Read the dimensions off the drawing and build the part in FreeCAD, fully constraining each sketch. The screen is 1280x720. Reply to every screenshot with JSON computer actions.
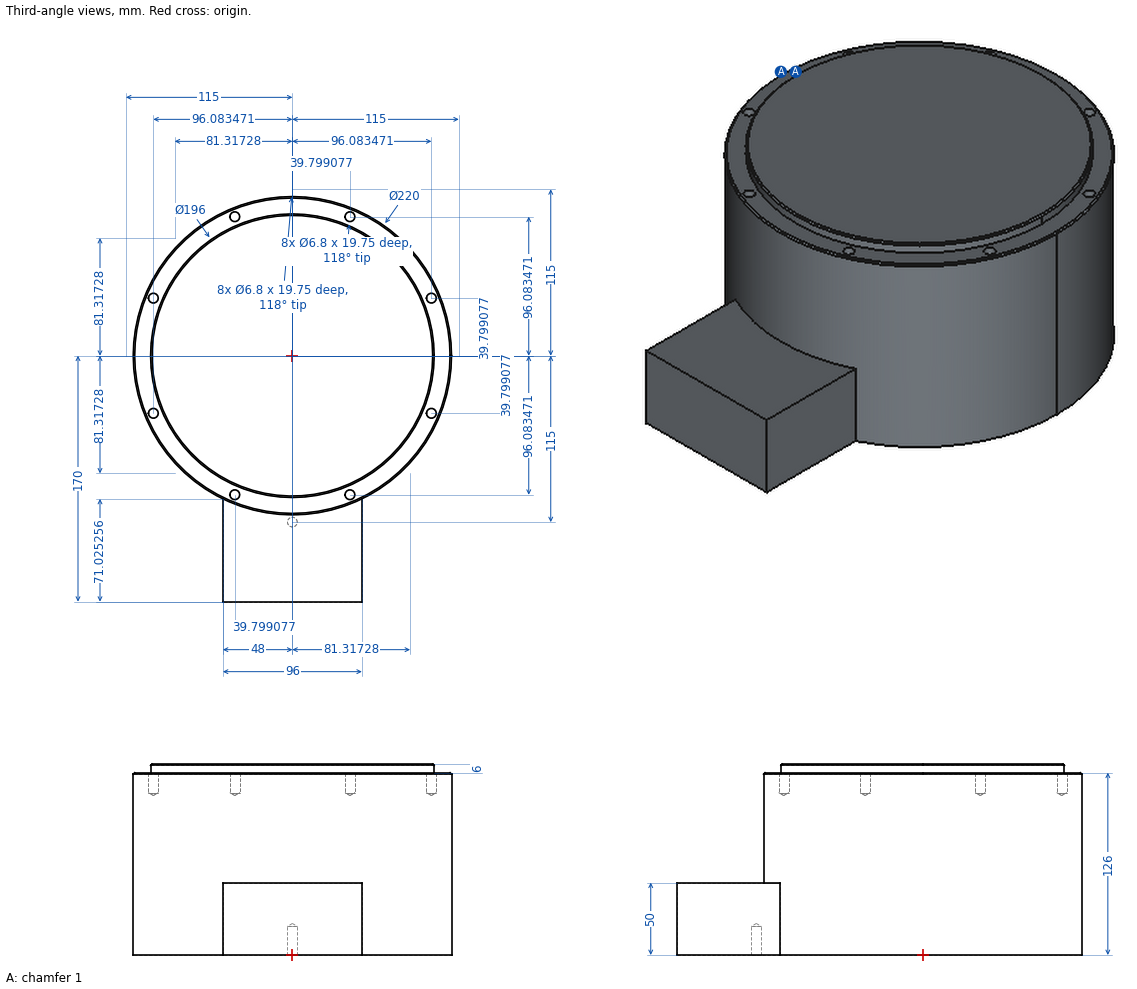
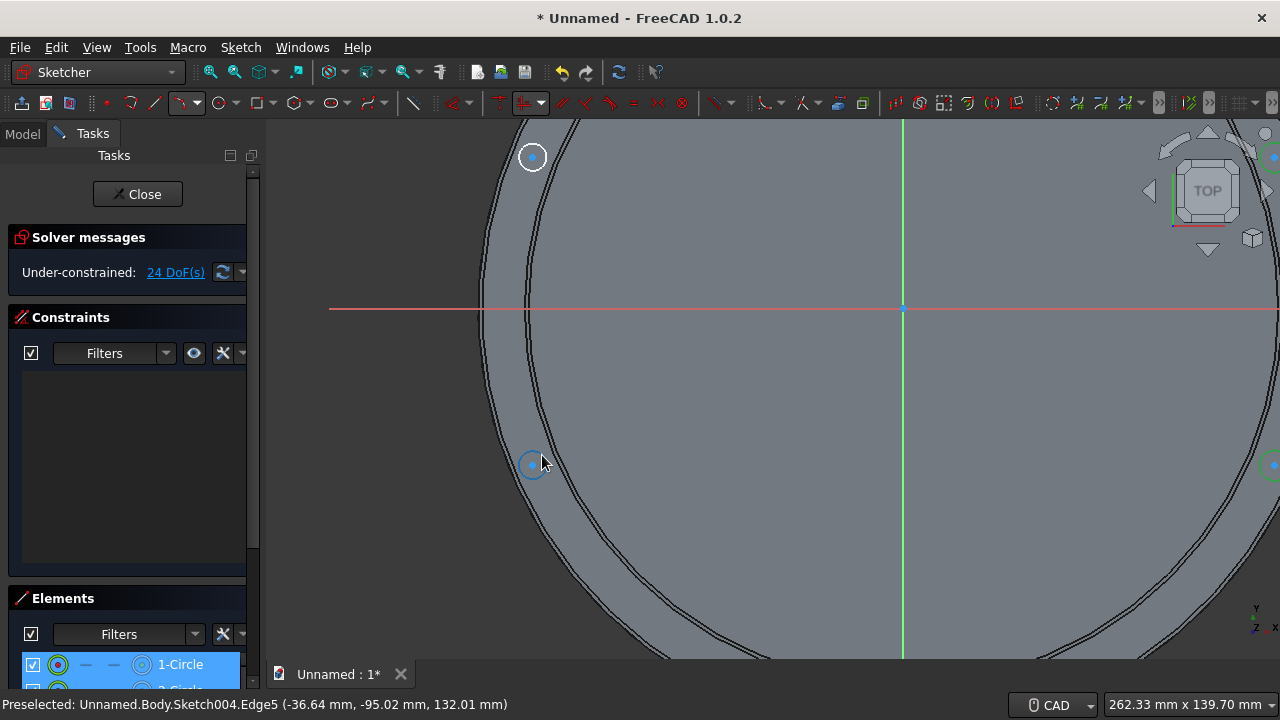
{"action": "left_click", "coordinate": [543, 455]}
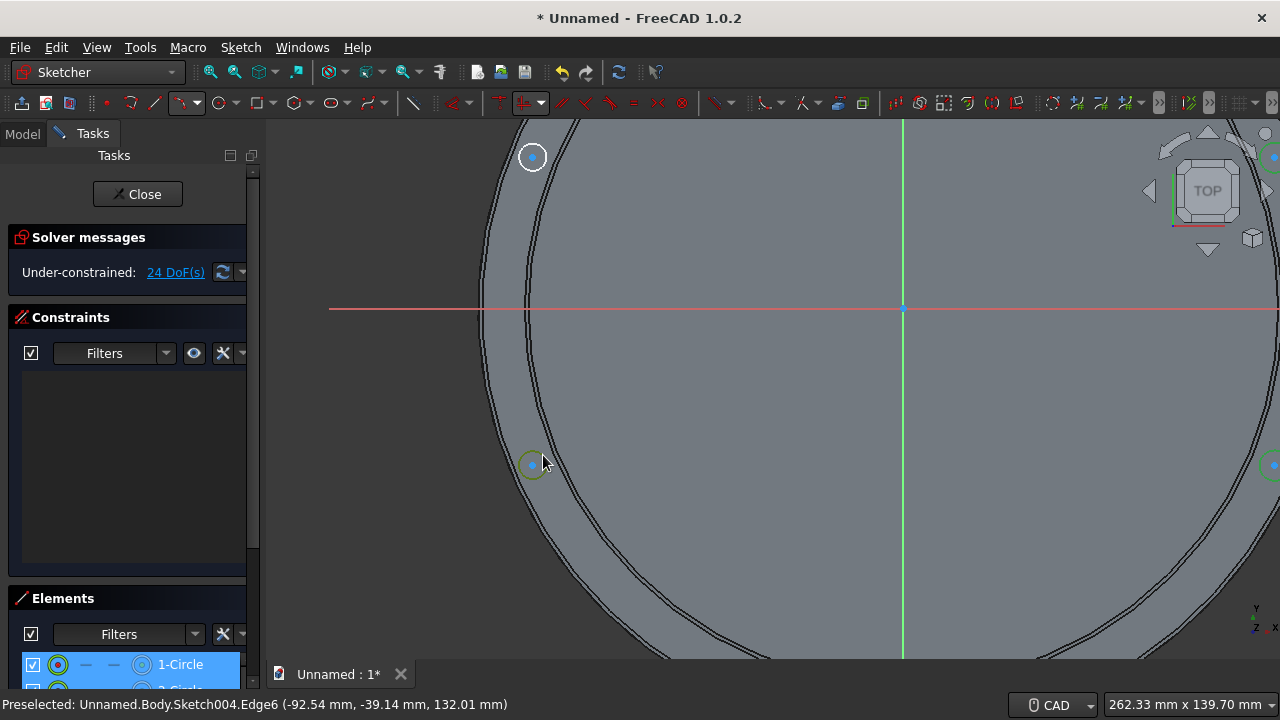
{"action": "left_click", "coordinate": [542, 148]}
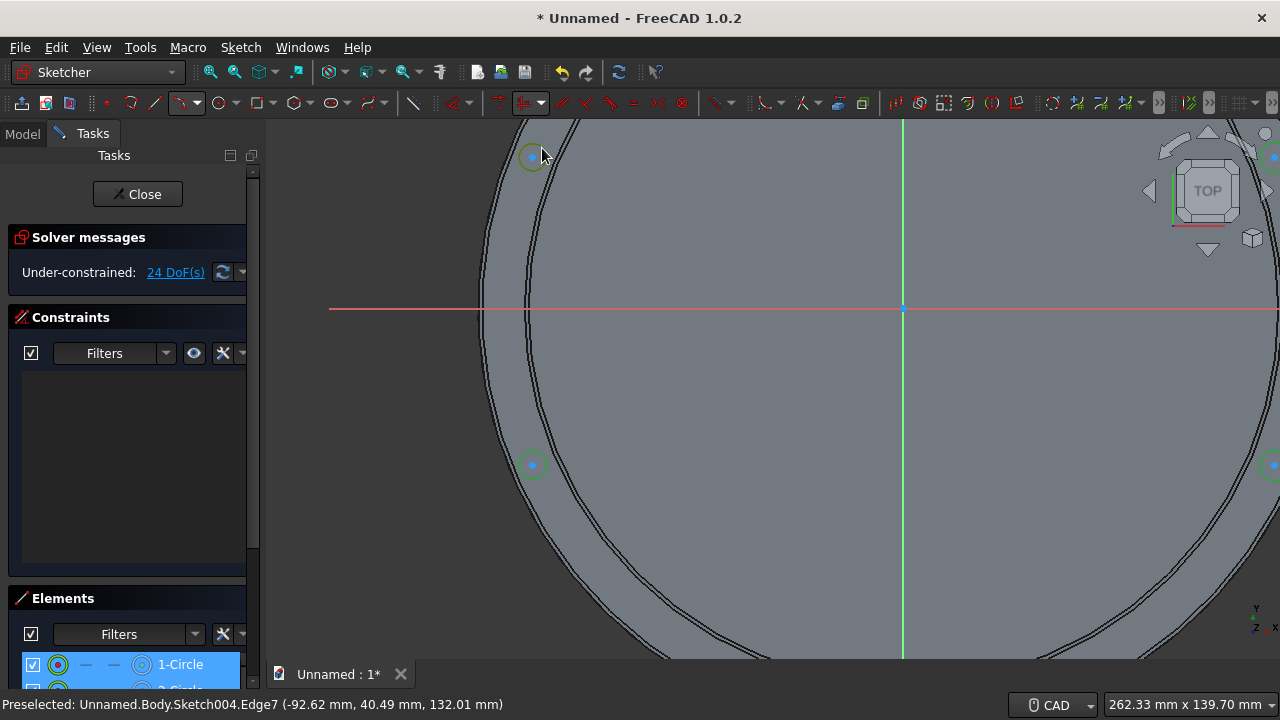
{"action": "scroll", "coordinate": [542, 454], "scroll_direction": "down", "scroll_amount": 4}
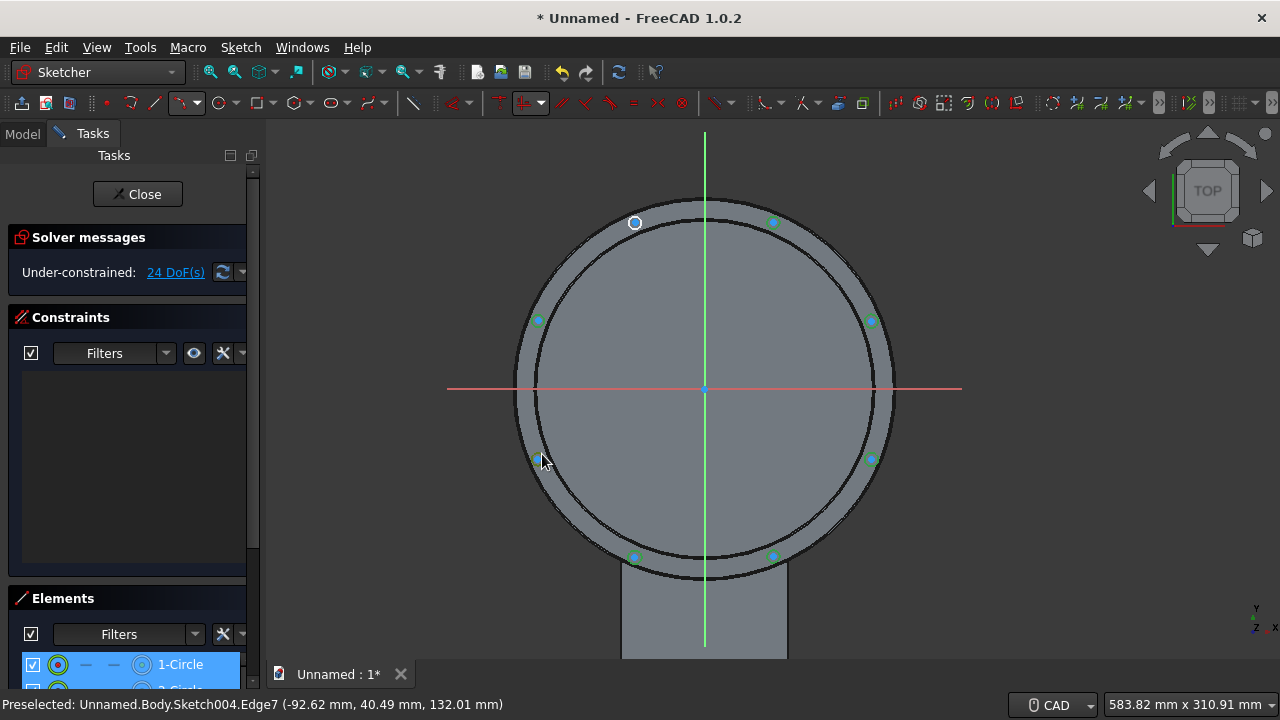
{"action": "scroll", "coordinate": [639, 218], "scroll_direction": "up", "scroll_amount": 4}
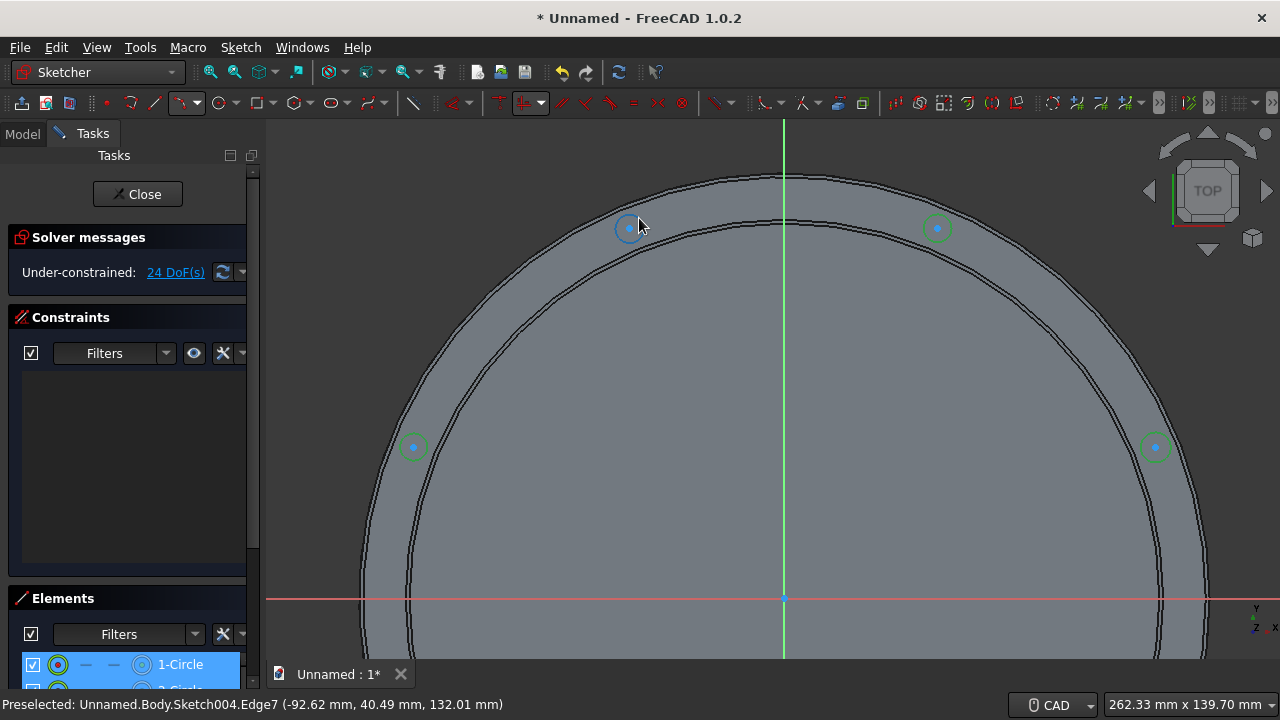
{"action": "left_click", "coordinate": [640, 219]}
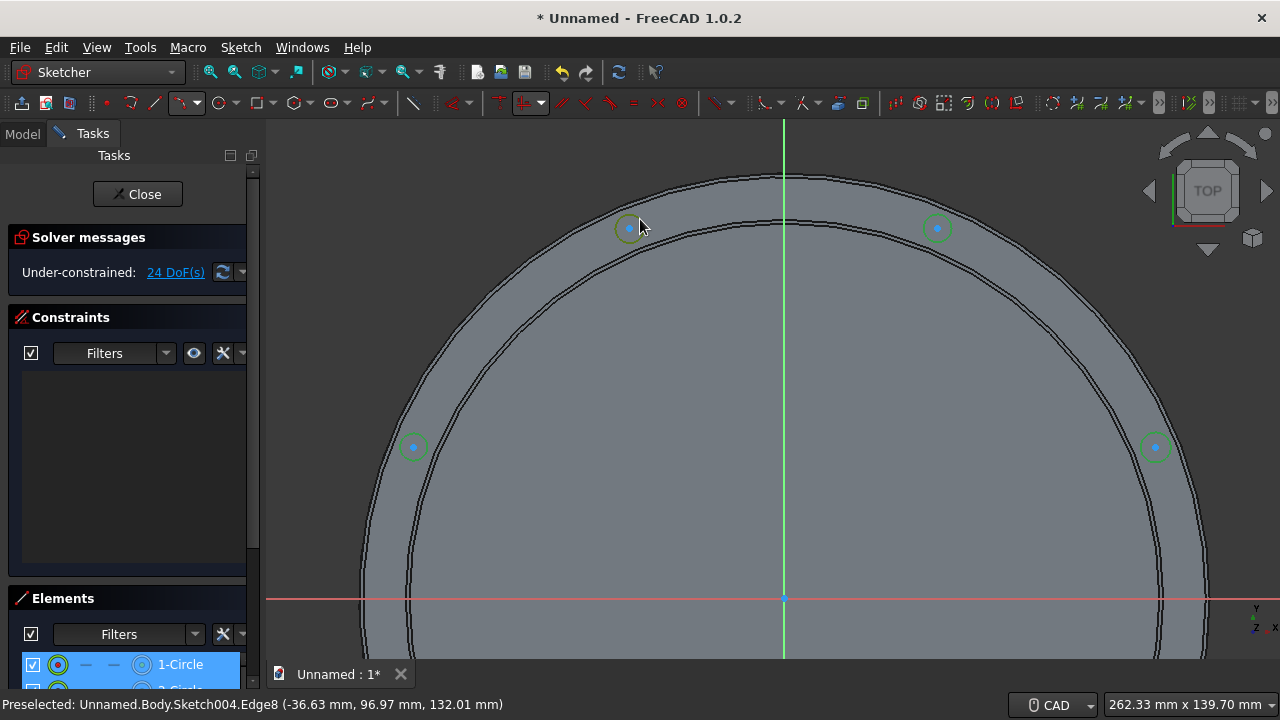
{"action": "left_click", "coordinate": [634, 104]}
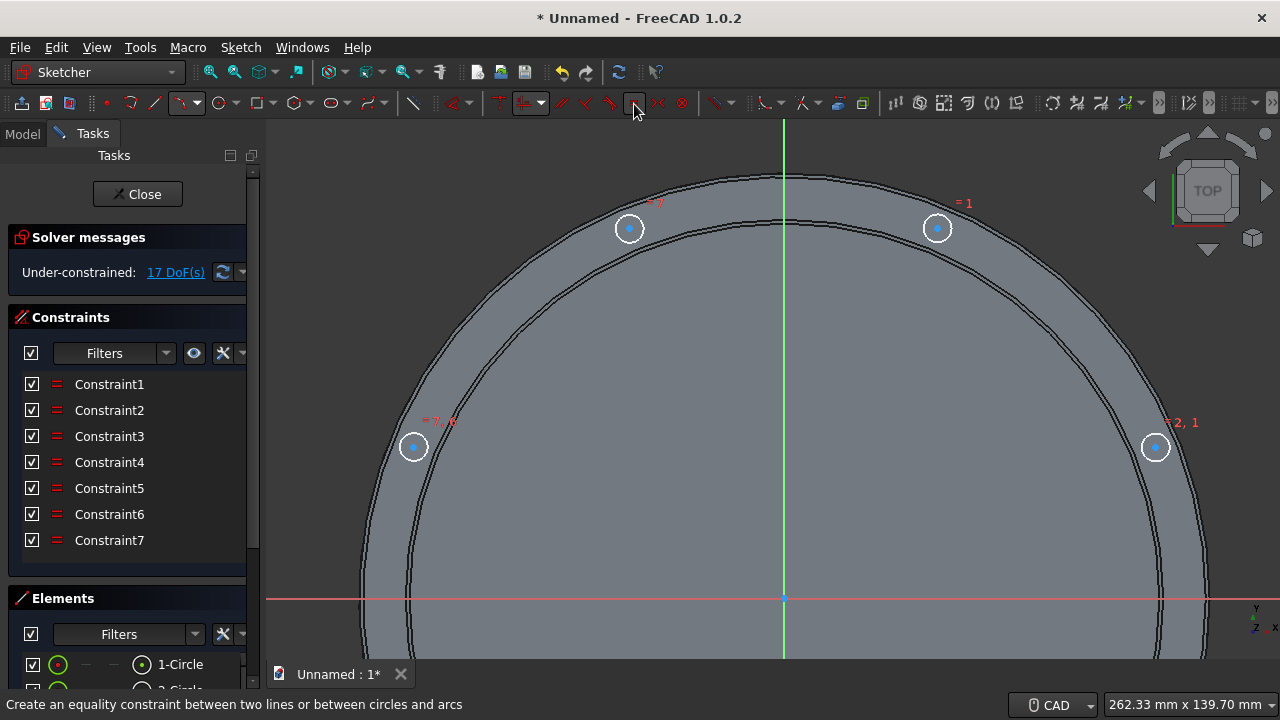
{"action": "scroll", "coordinate": [639, 218], "scroll_direction": "down", "scroll_amount": 4}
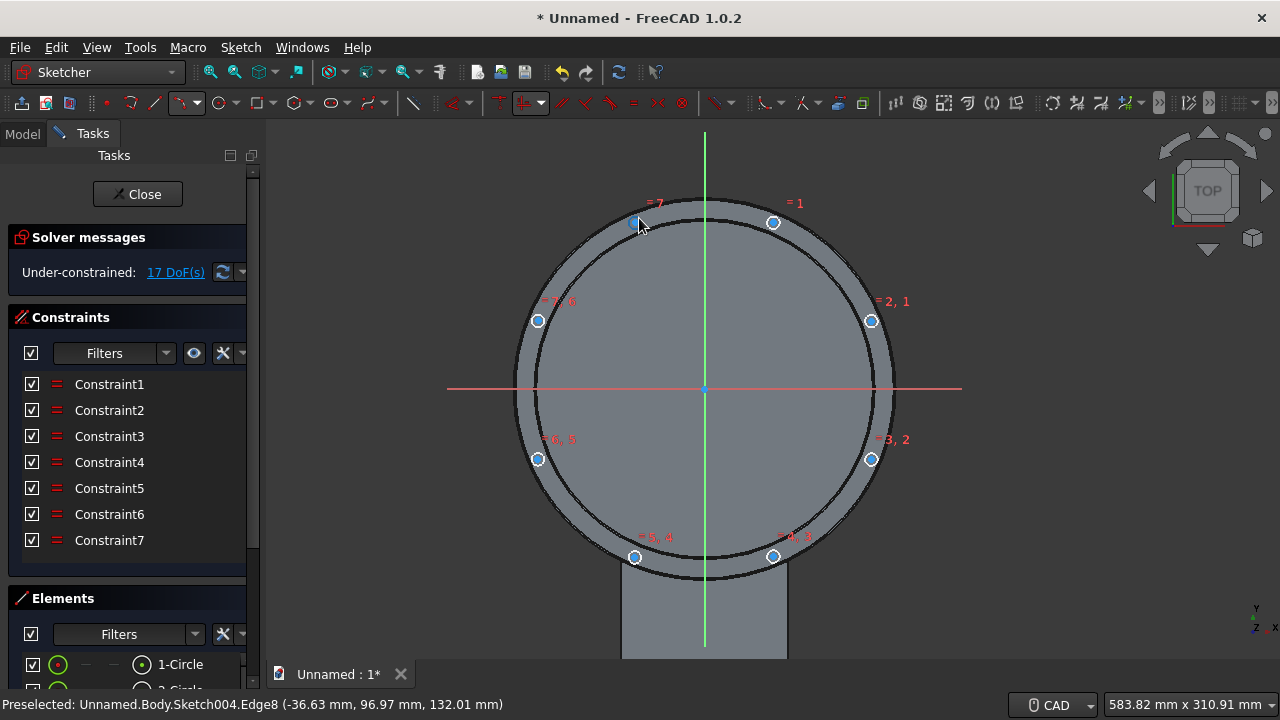
{"action": "left_click", "coordinate": [871, 321]}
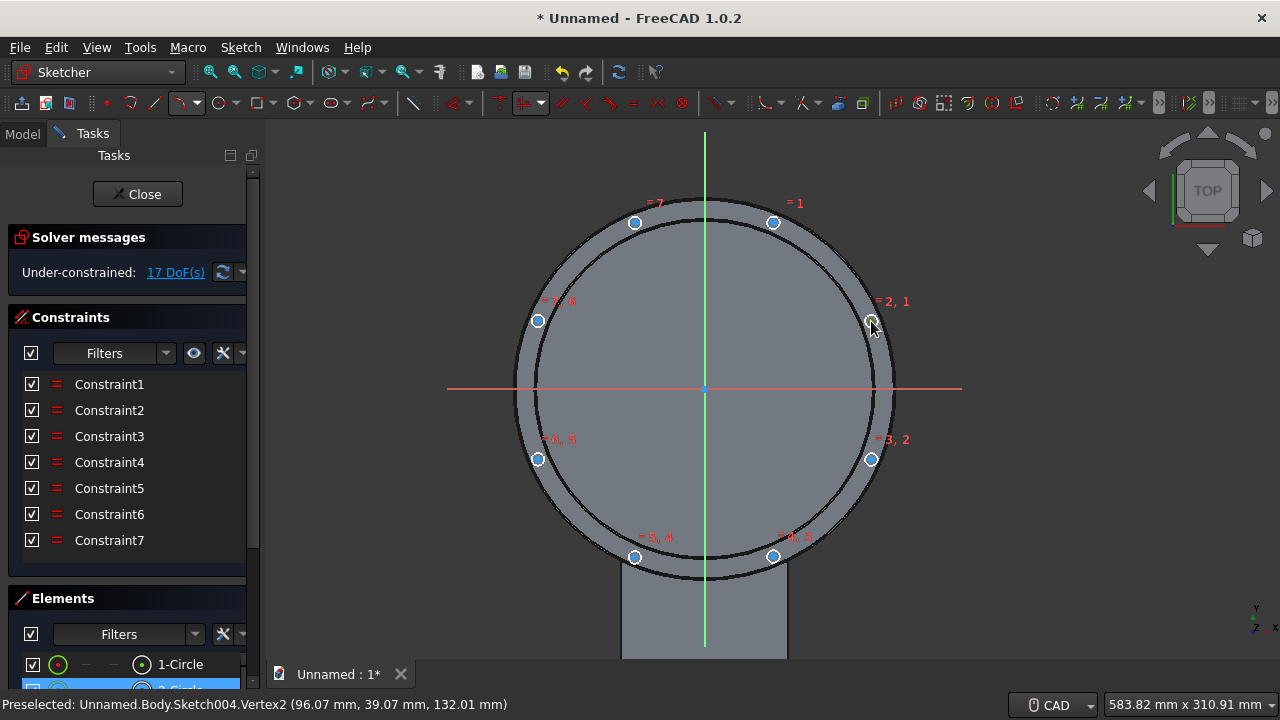
{"action": "left_click", "coordinate": [871, 460]}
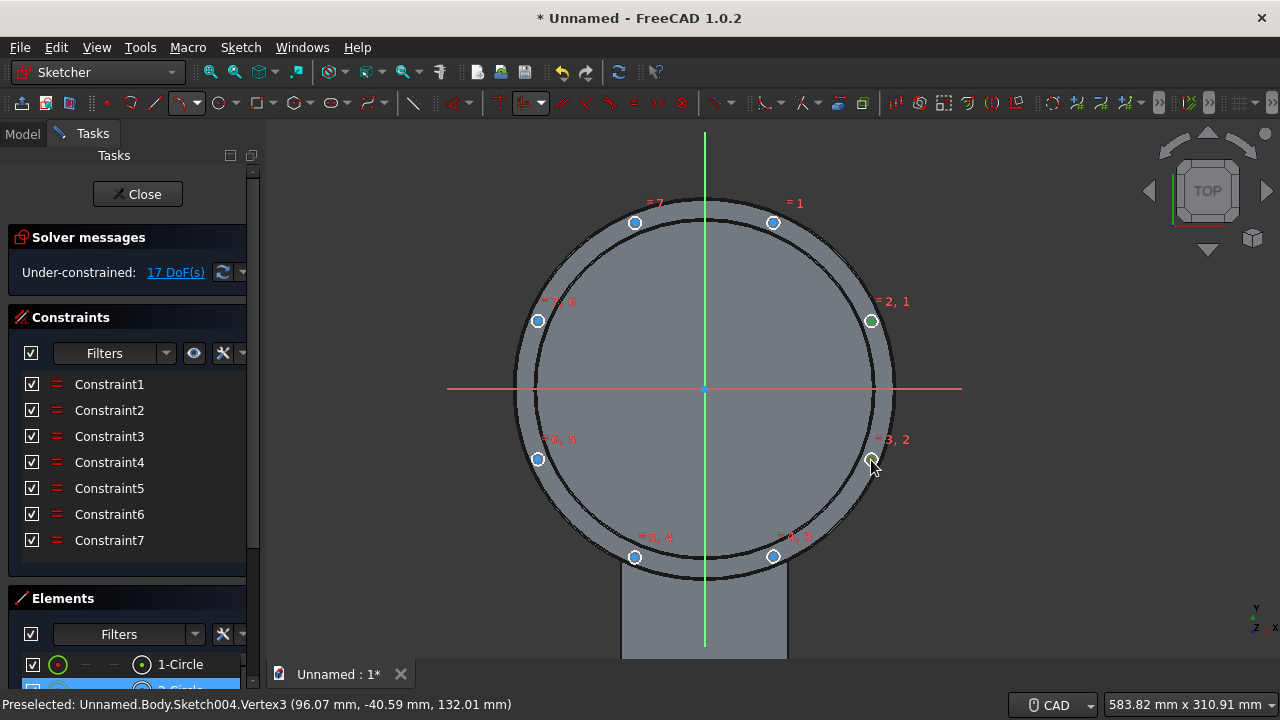
{"action": "key", "text": "v"}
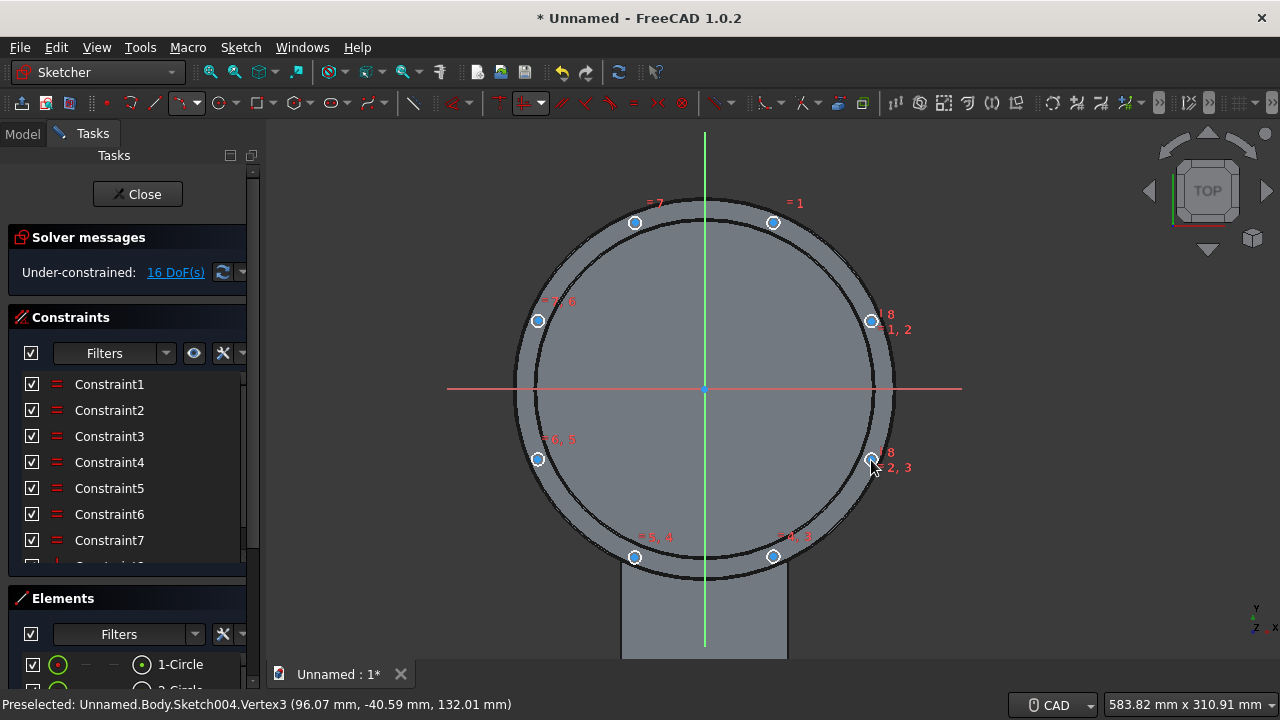
{"action": "left_click", "coordinate": [773, 223]}